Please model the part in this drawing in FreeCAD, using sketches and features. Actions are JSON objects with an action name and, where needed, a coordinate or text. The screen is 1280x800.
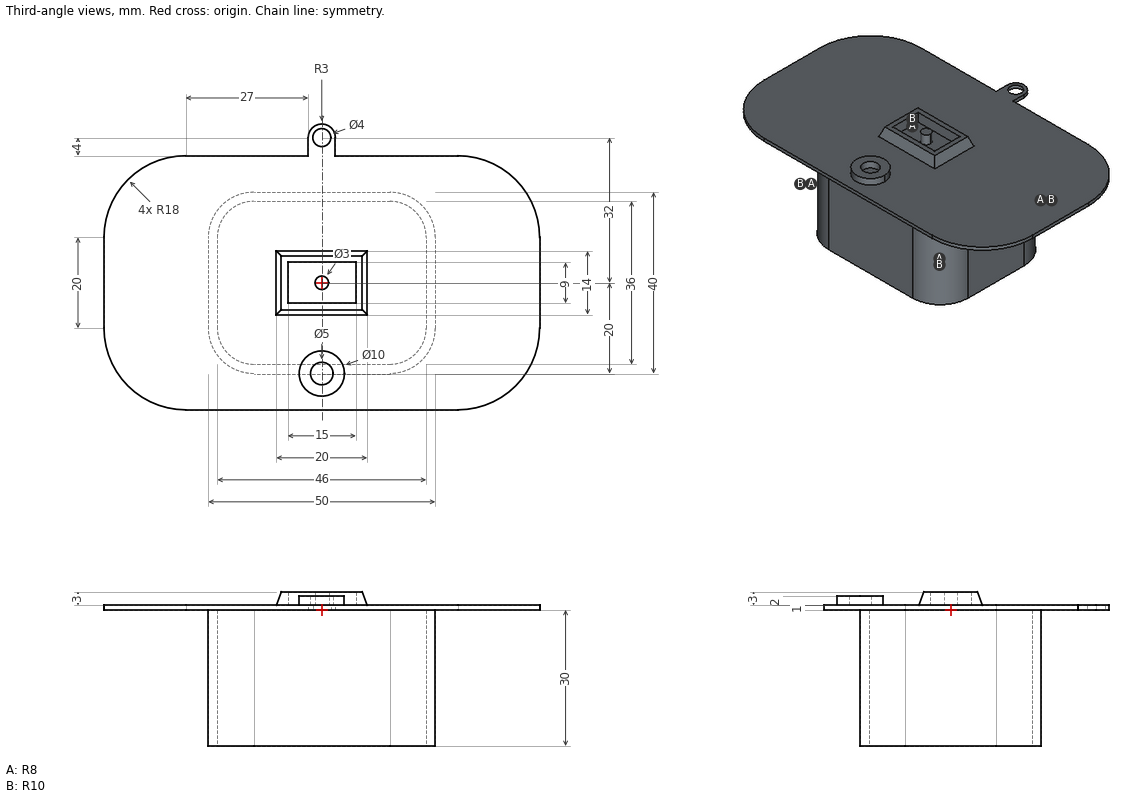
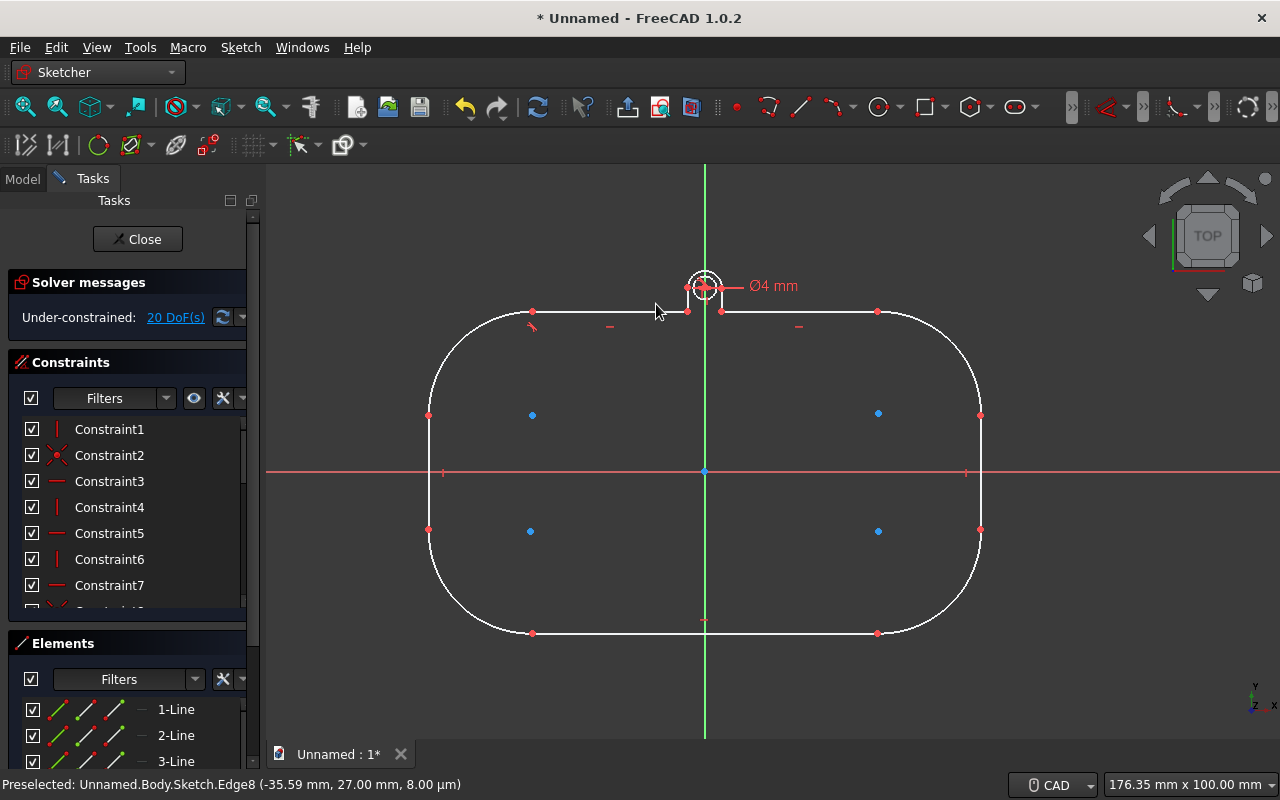
{"action": "left_click", "coordinate": [429, 450]}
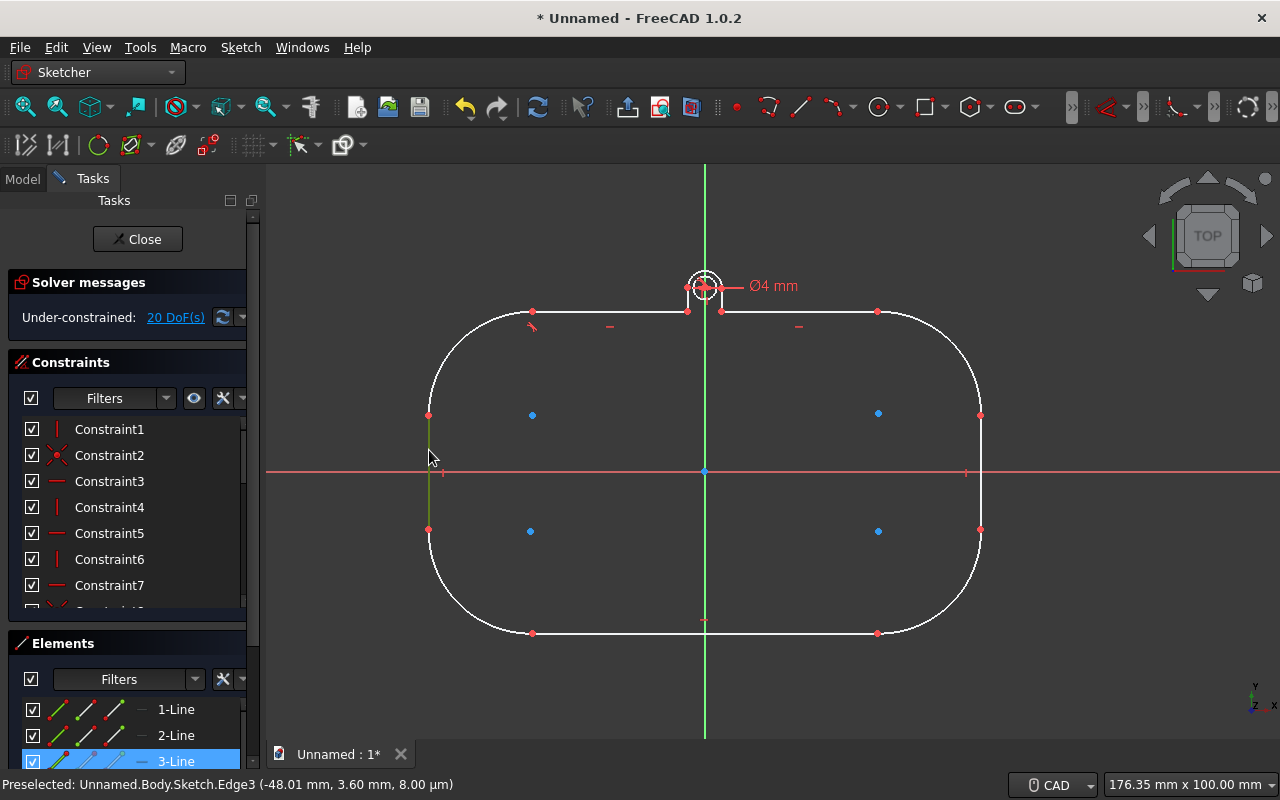
{"action": "left_click", "coordinate": [485, 323]}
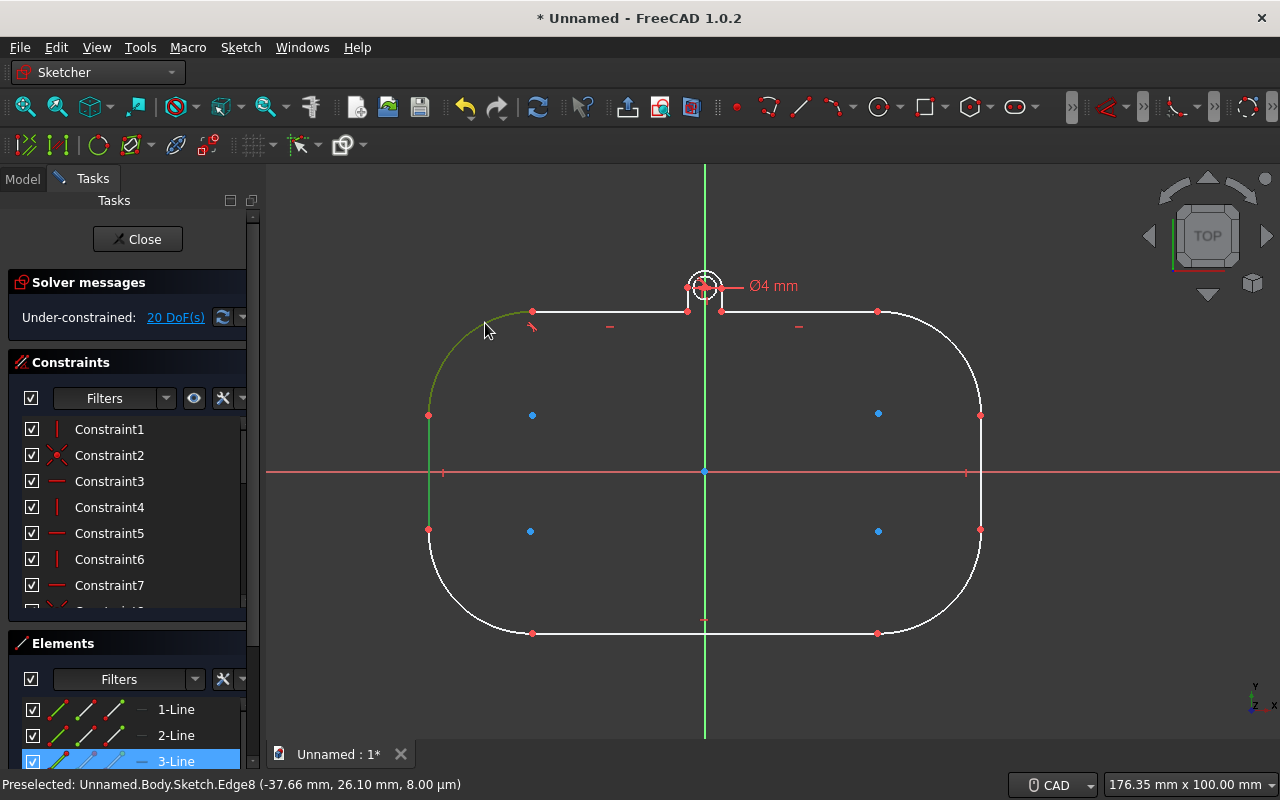
{"action": "key", "text": "t"}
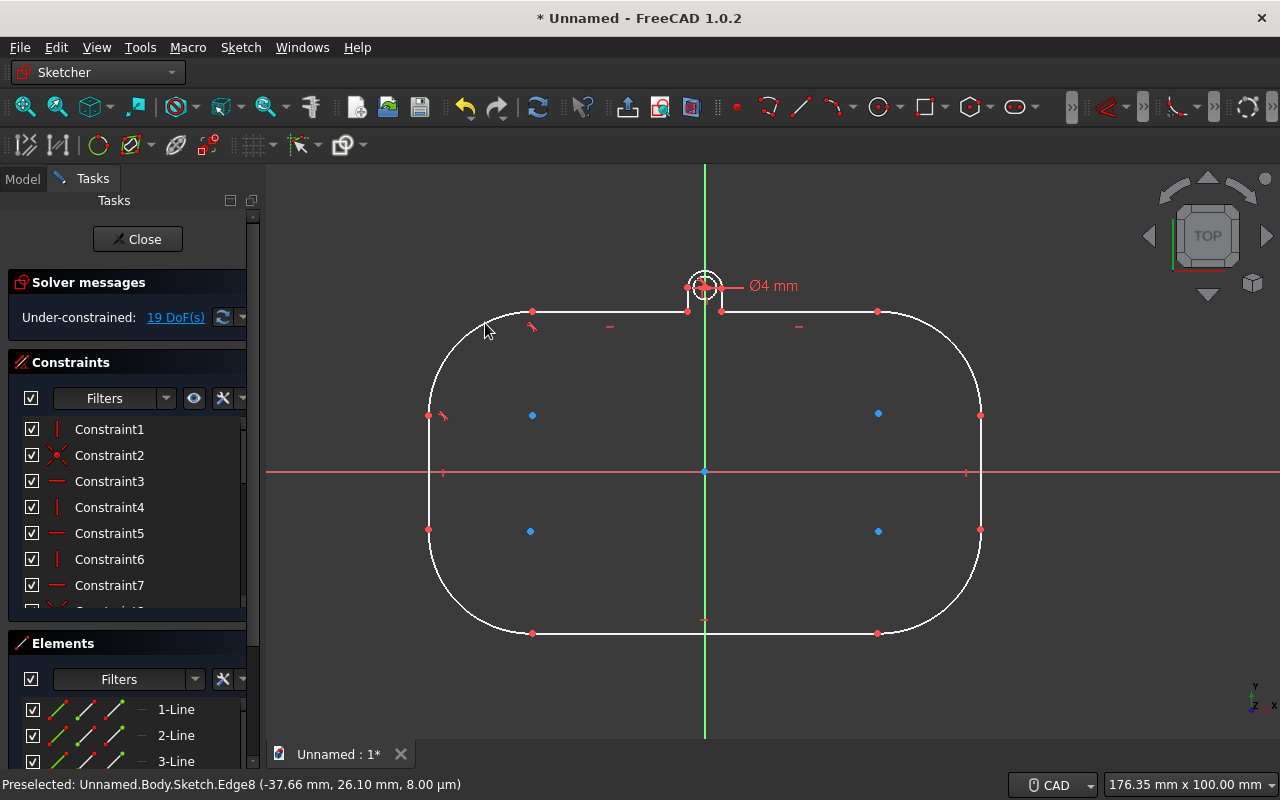
{"action": "left_click", "coordinate": [429, 450]}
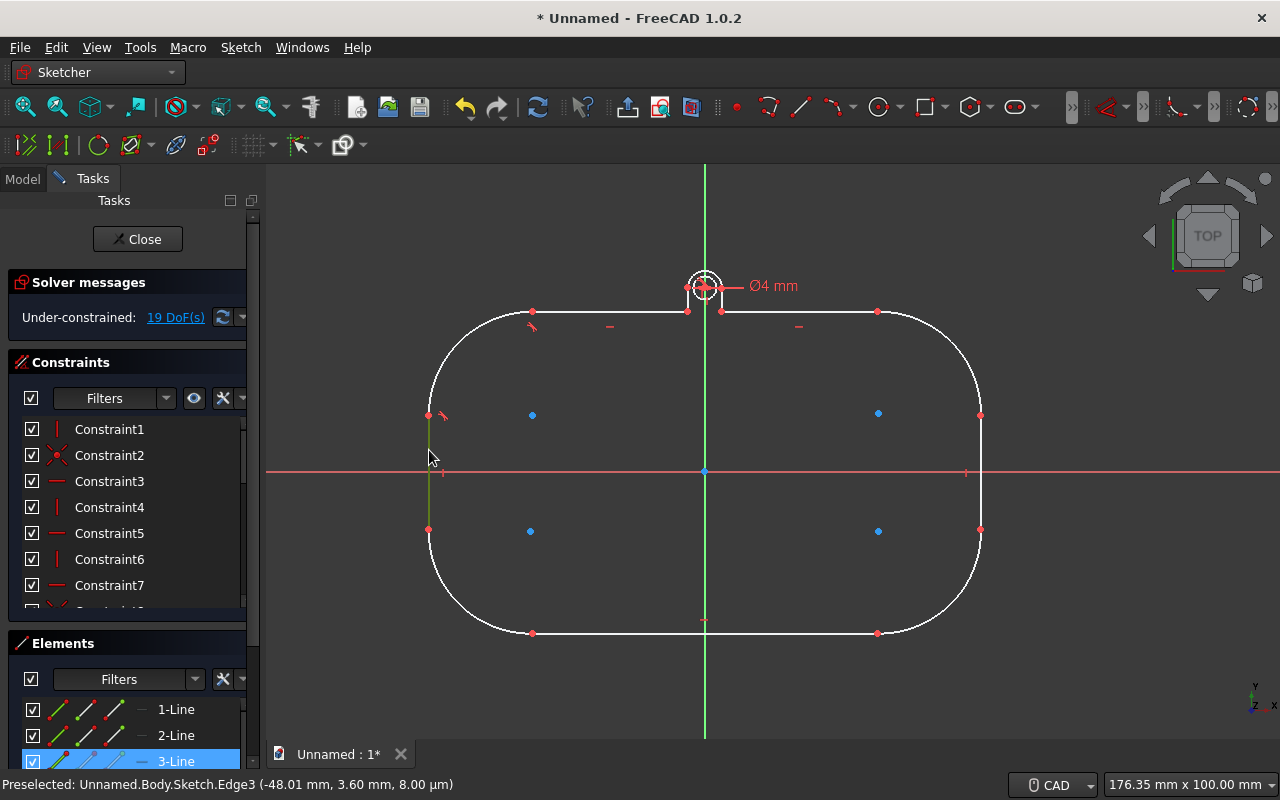
{"action": "left_click", "coordinate": [440, 577]}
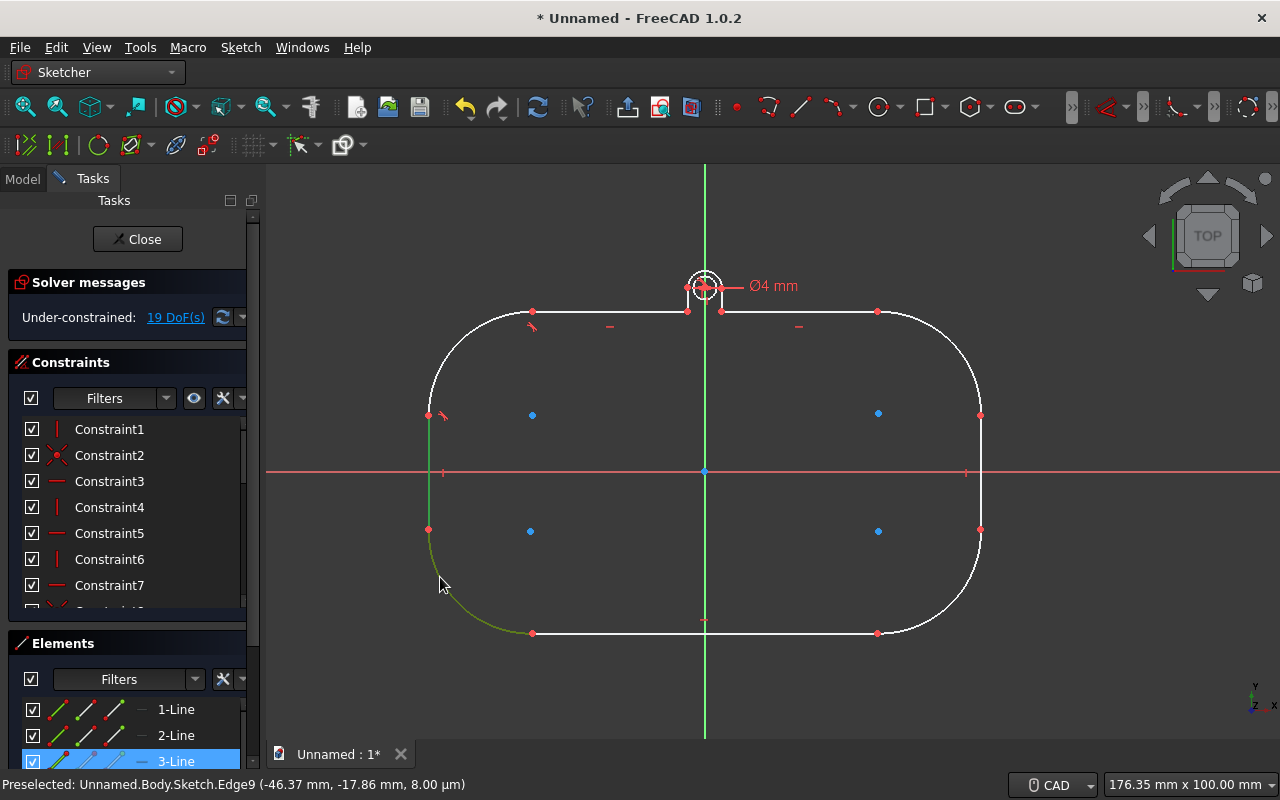
{"action": "key", "text": "t"}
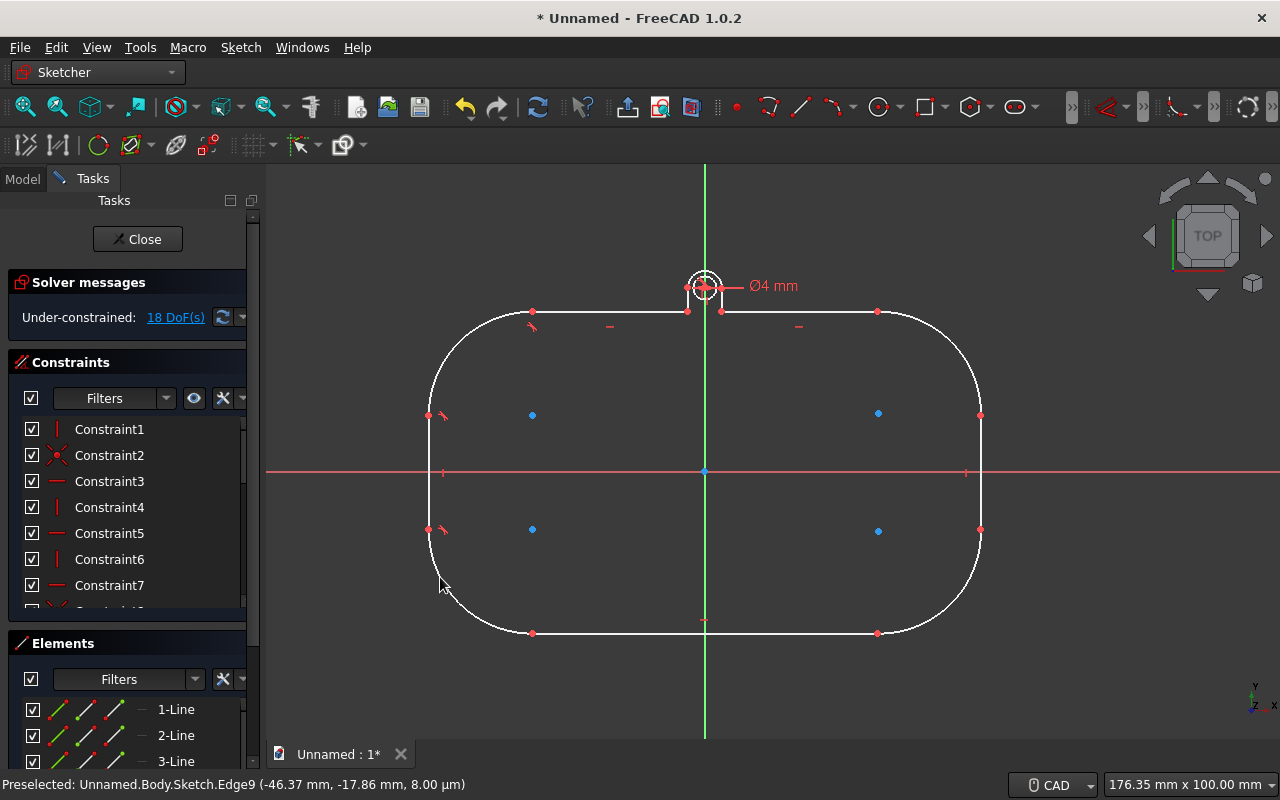
{"action": "left_click", "coordinate": [636, 634]}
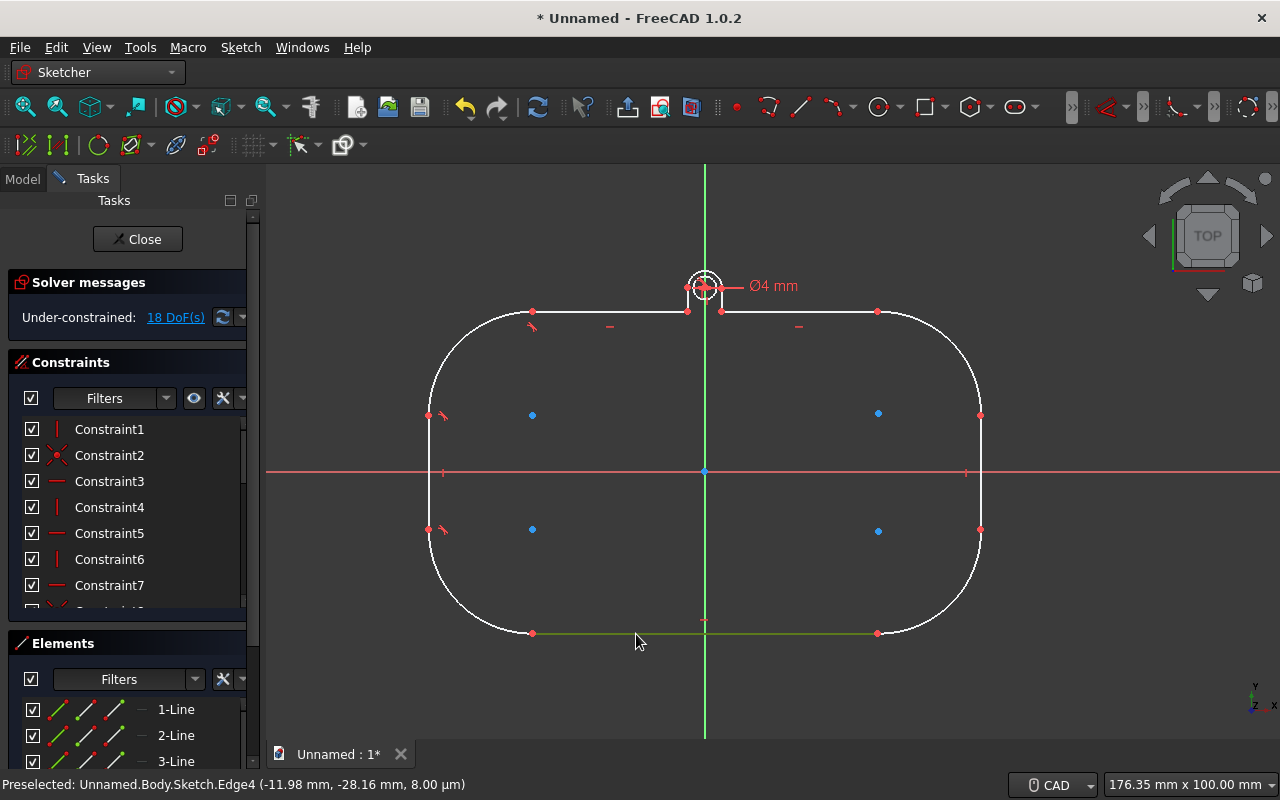
{"action": "left_click", "coordinate": [440, 577]}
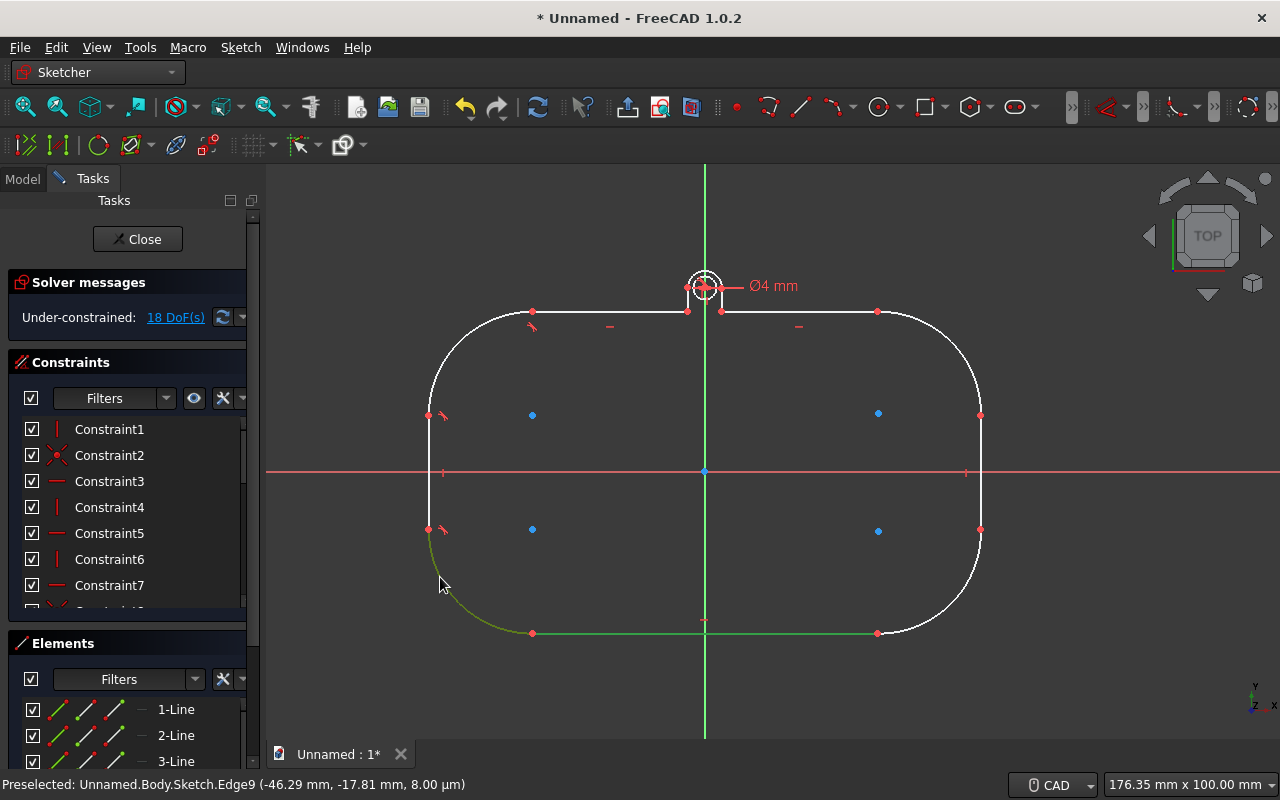
{"action": "key", "text": "t"}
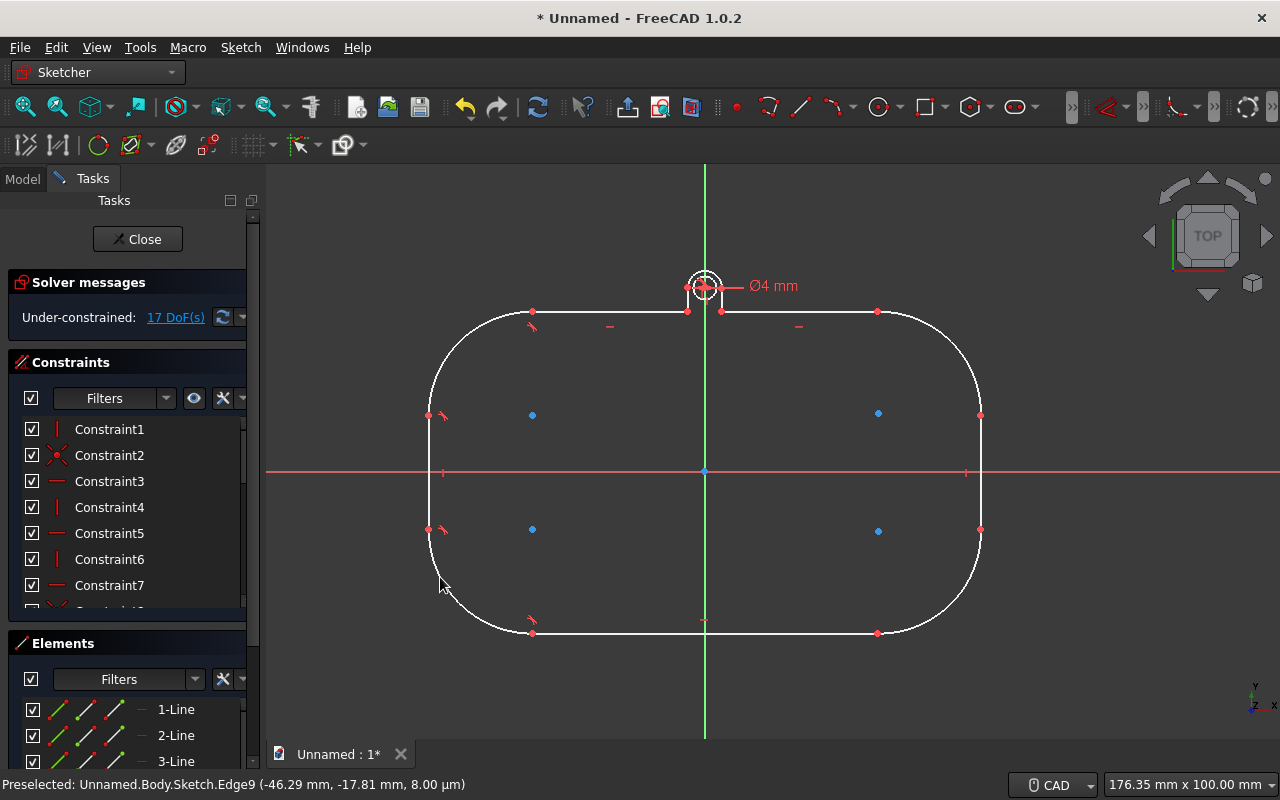
{"action": "left_click", "coordinate": [636, 634]}